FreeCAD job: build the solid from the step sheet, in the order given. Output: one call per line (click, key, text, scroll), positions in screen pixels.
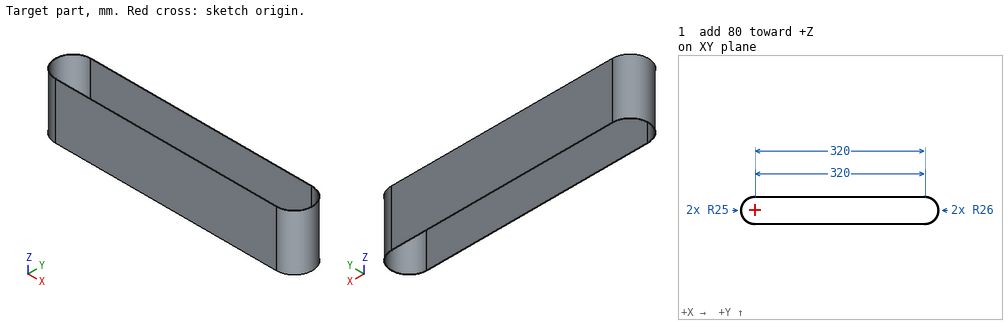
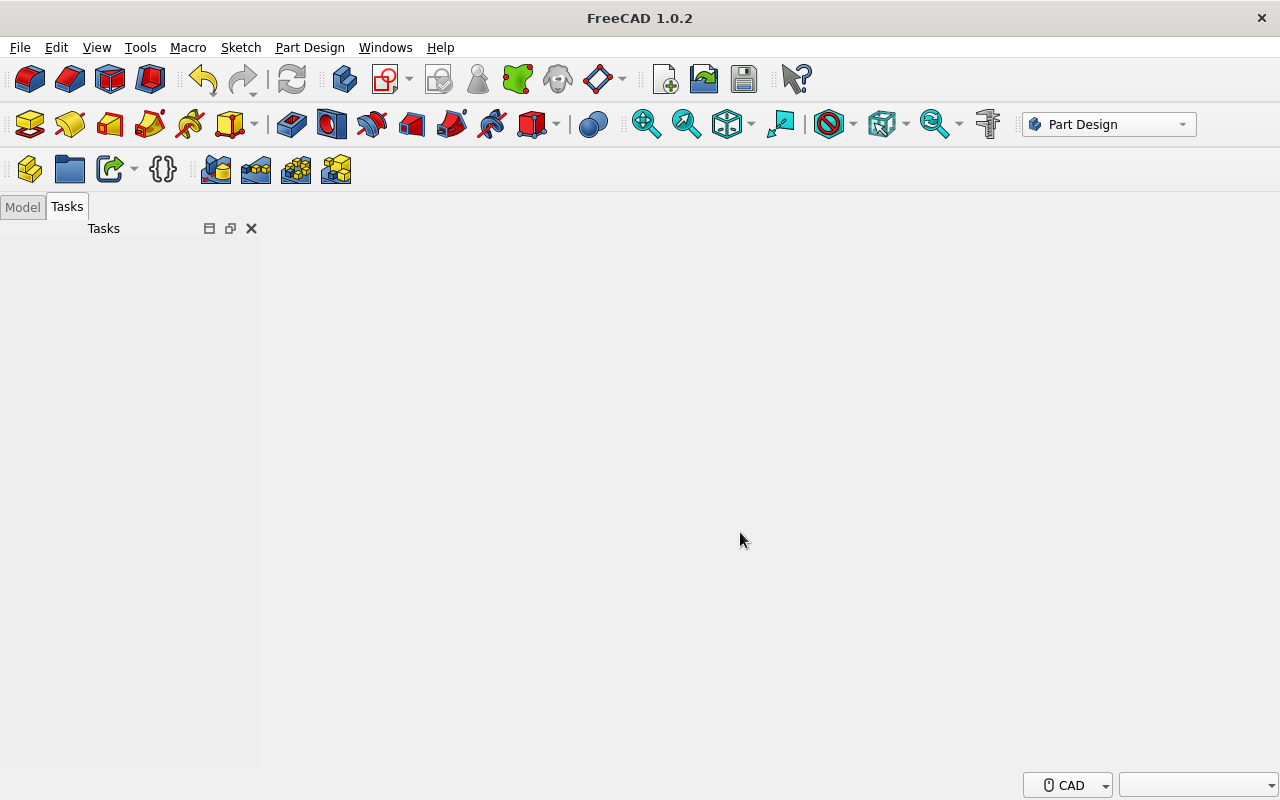
click(664, 80)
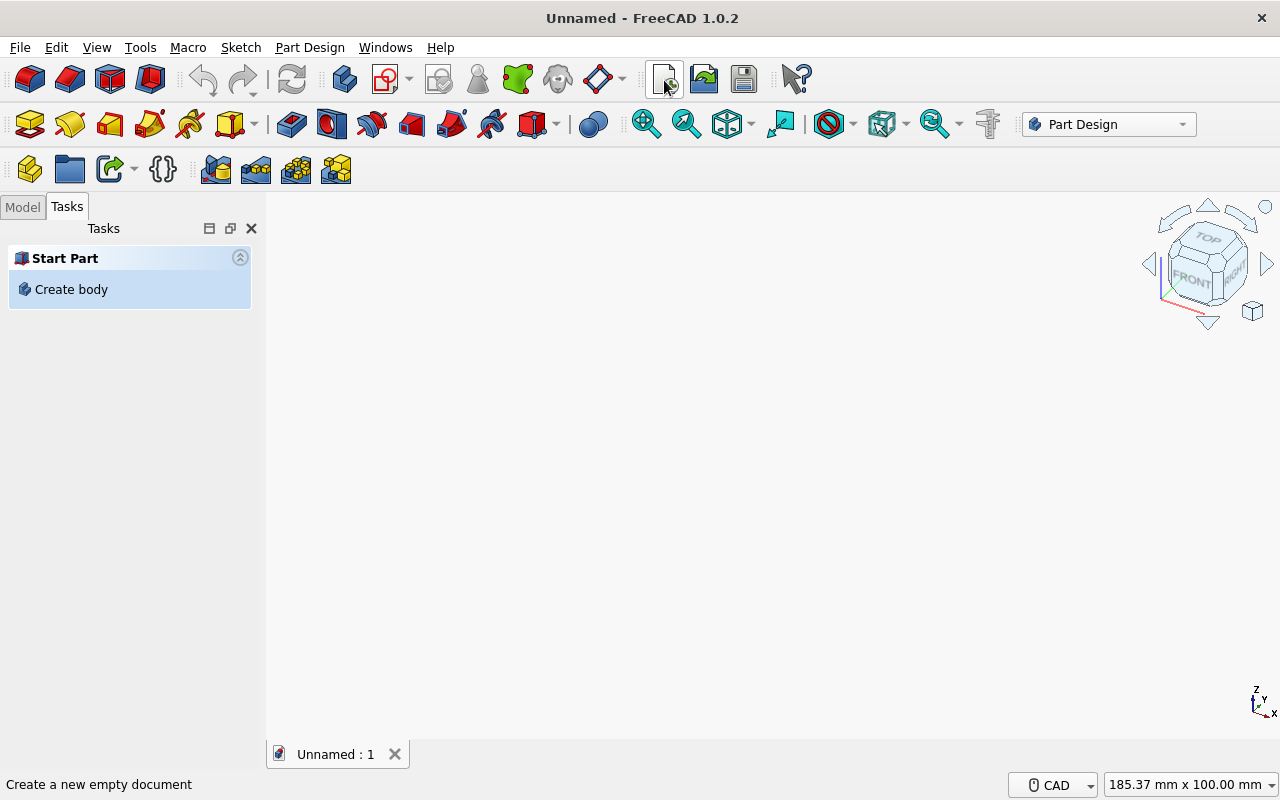
click(386, 80)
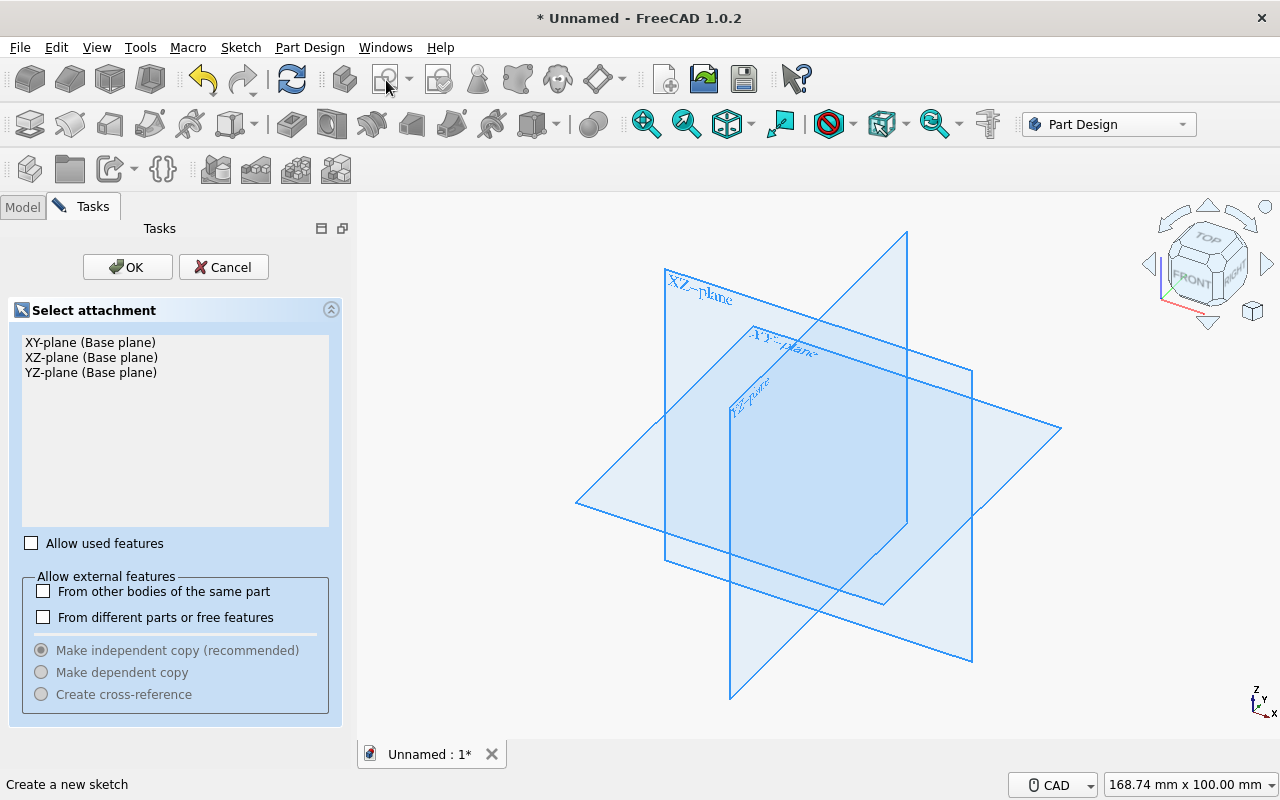
click(82, 342)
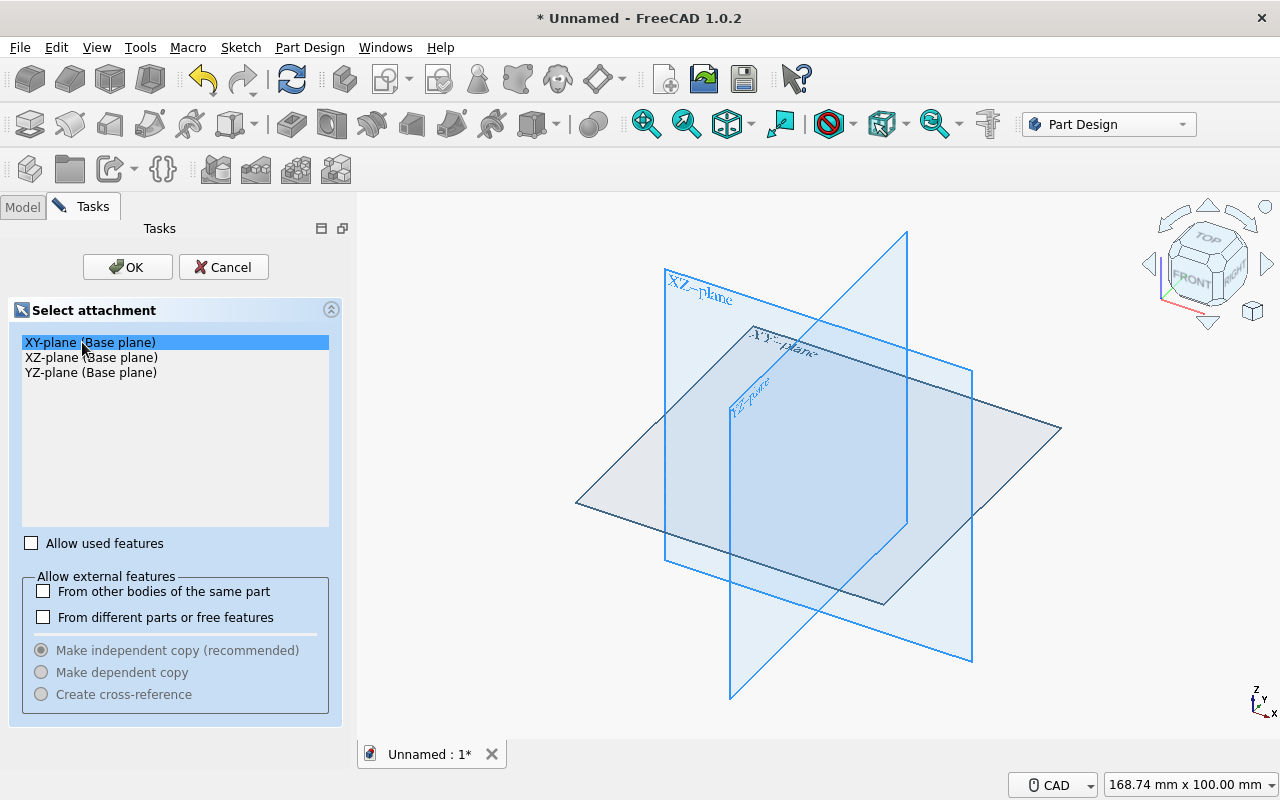
click(128, 267)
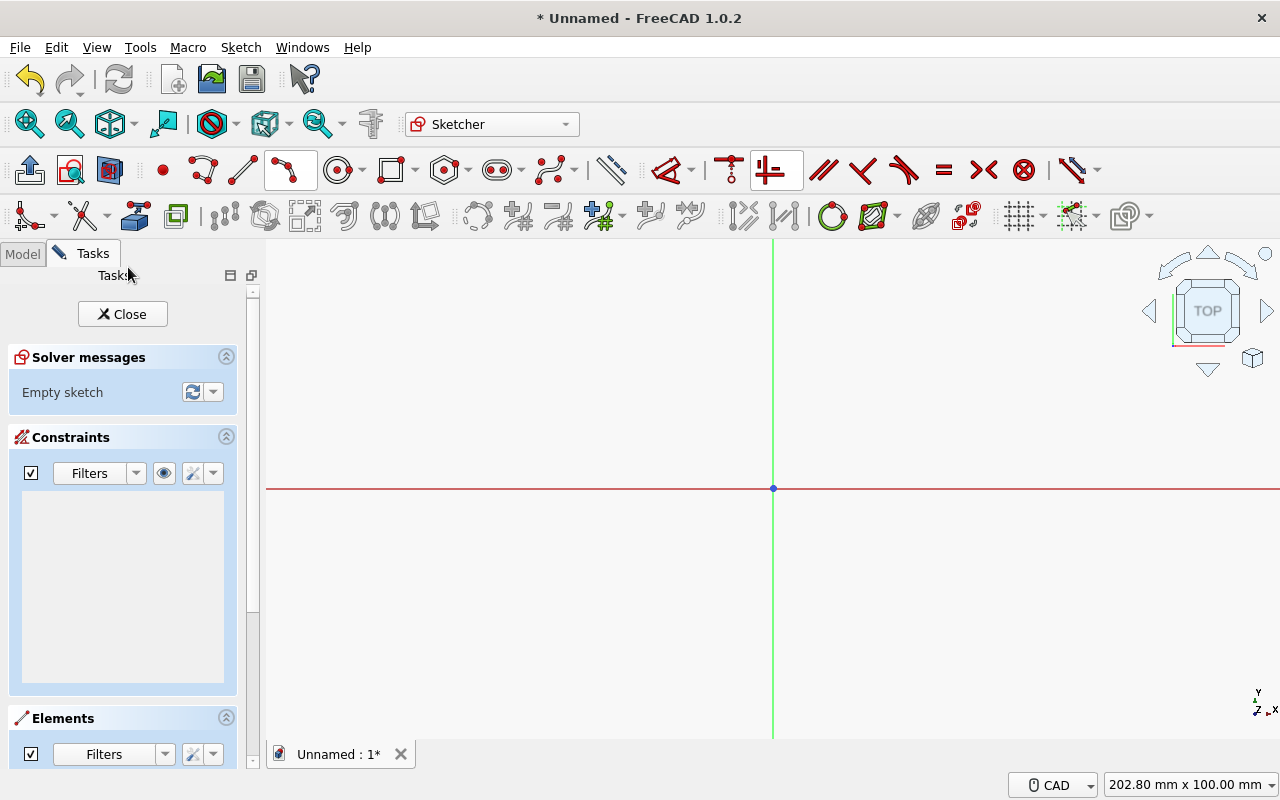
scroll(330, 489, down, 6)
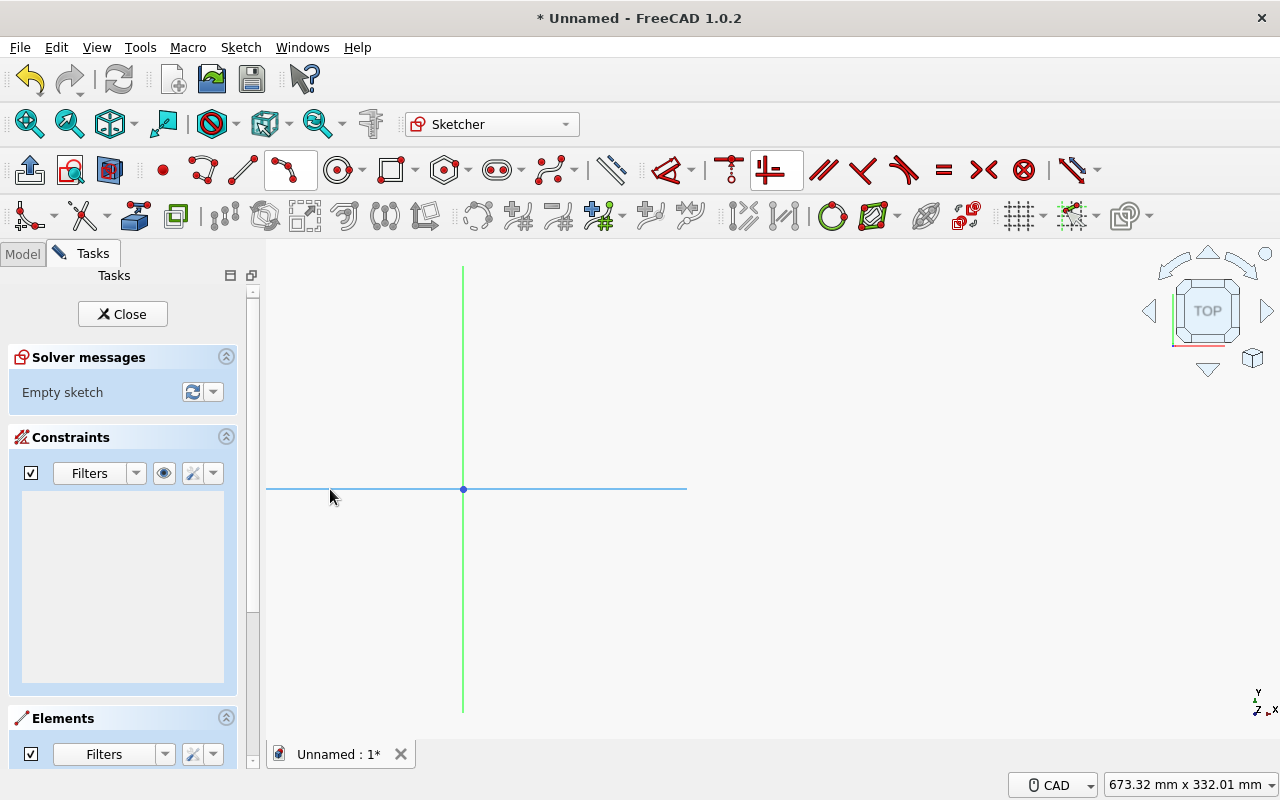
click(498, 170)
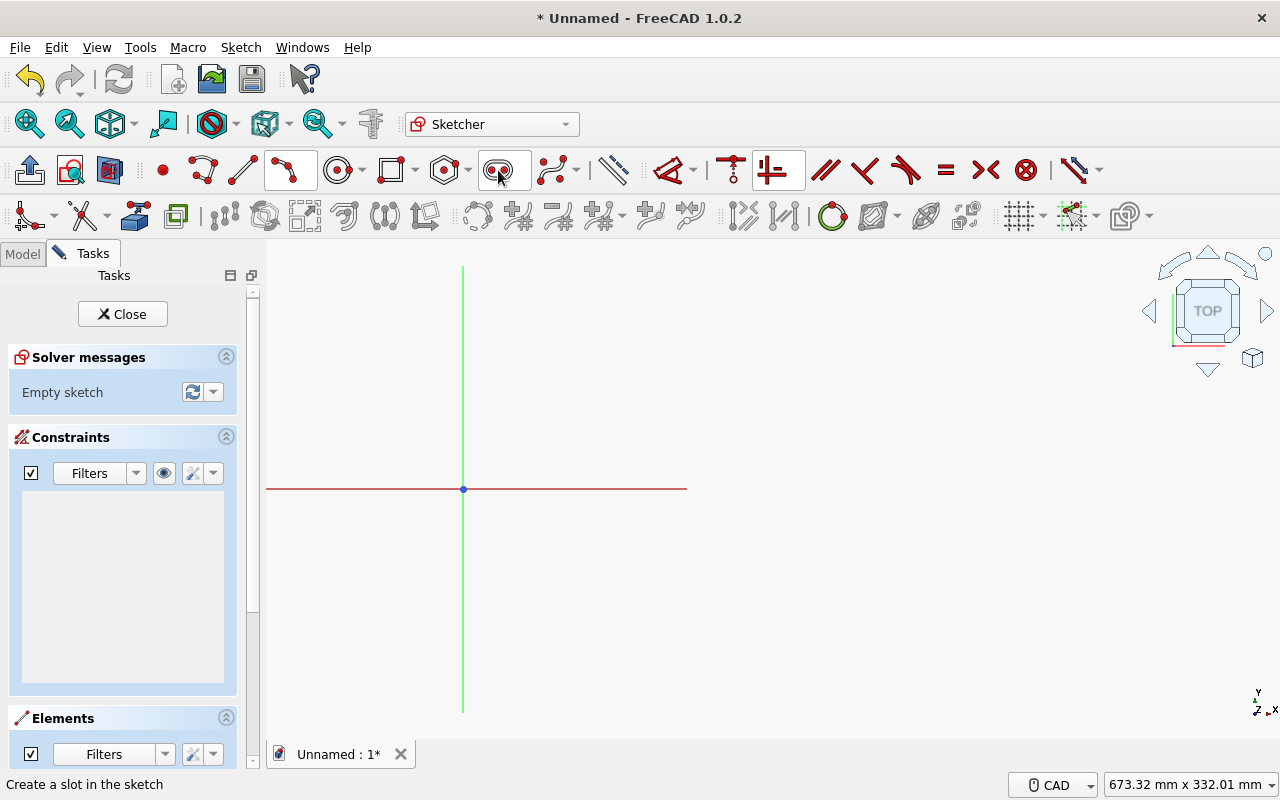
click(463, 489)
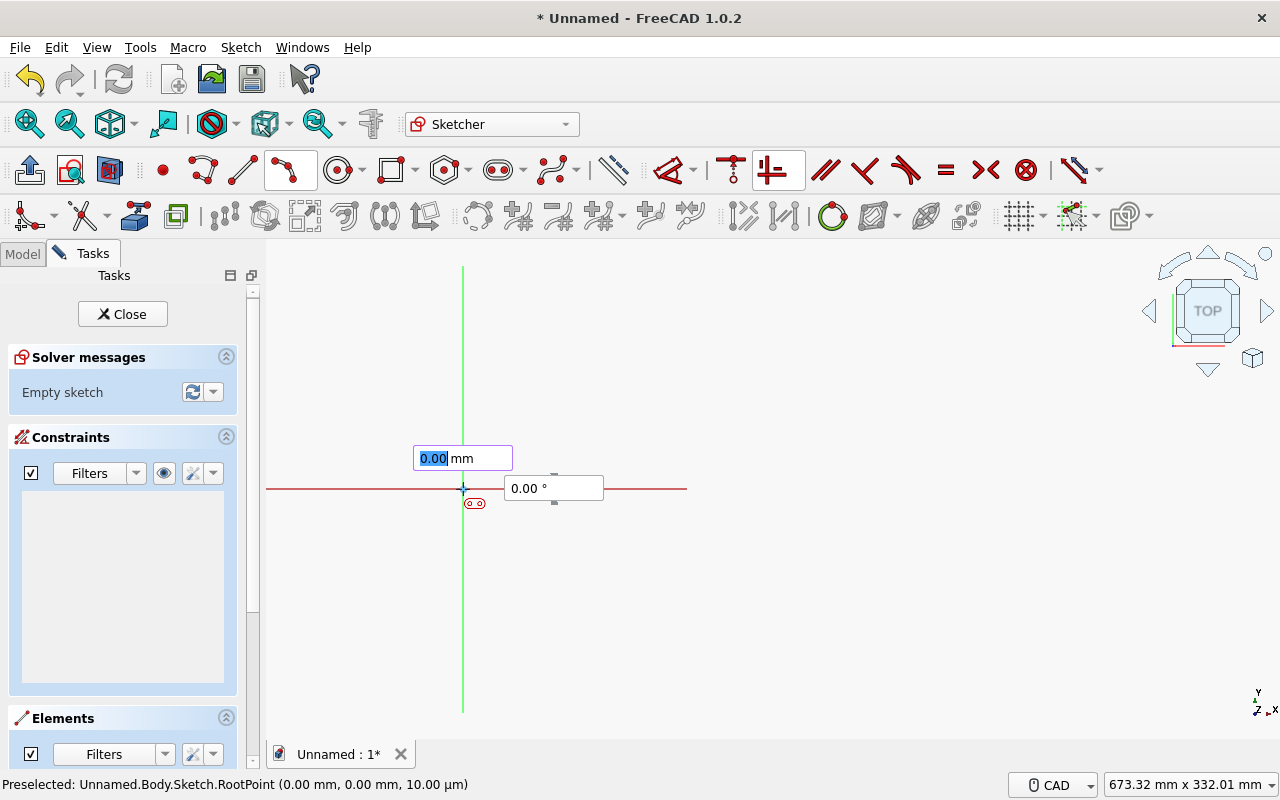
click(945, 480)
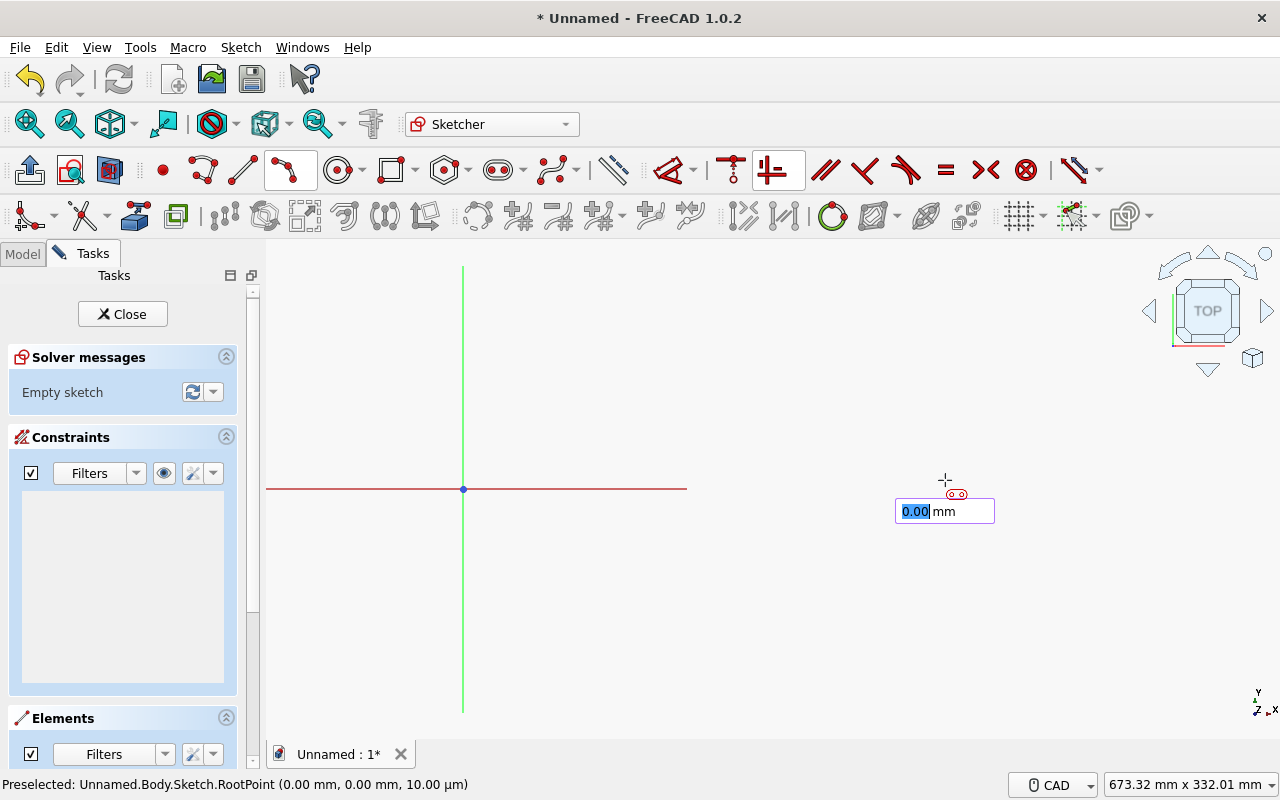
click(704, 529)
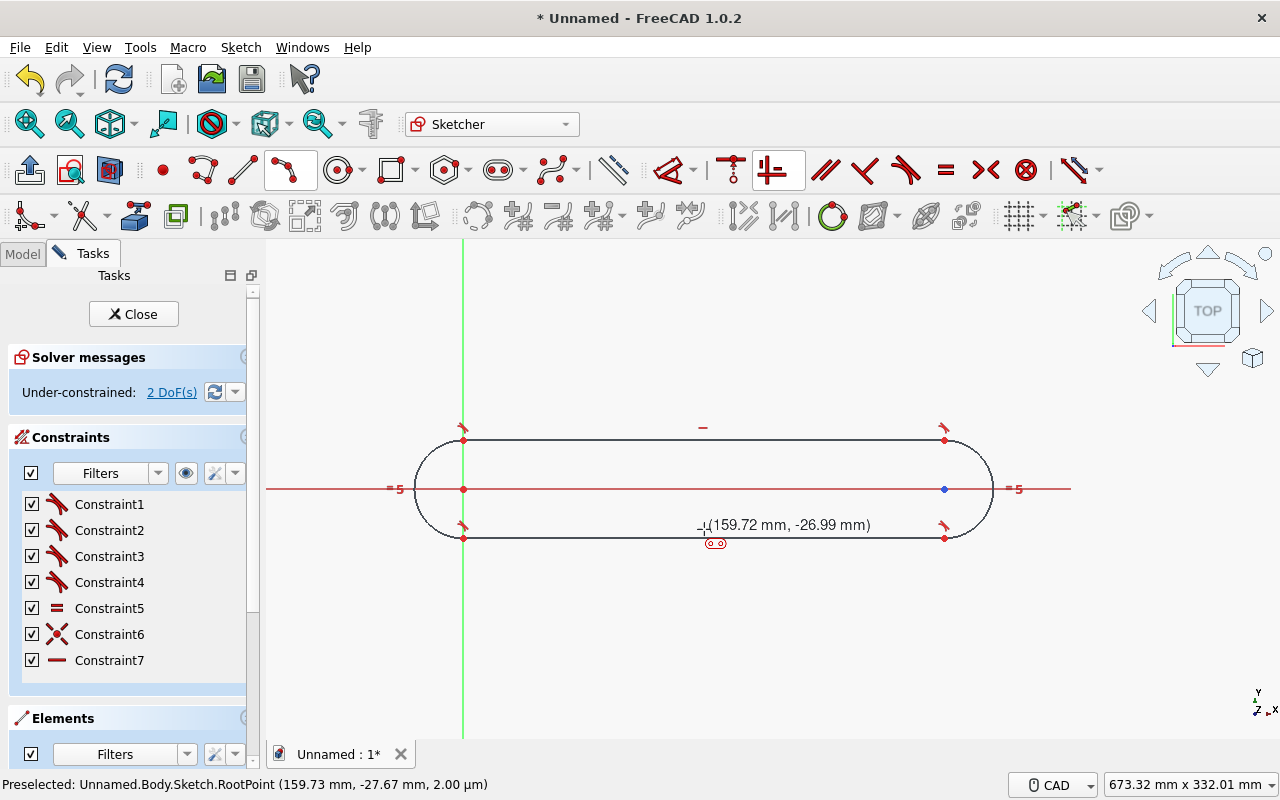
click(463, 489)